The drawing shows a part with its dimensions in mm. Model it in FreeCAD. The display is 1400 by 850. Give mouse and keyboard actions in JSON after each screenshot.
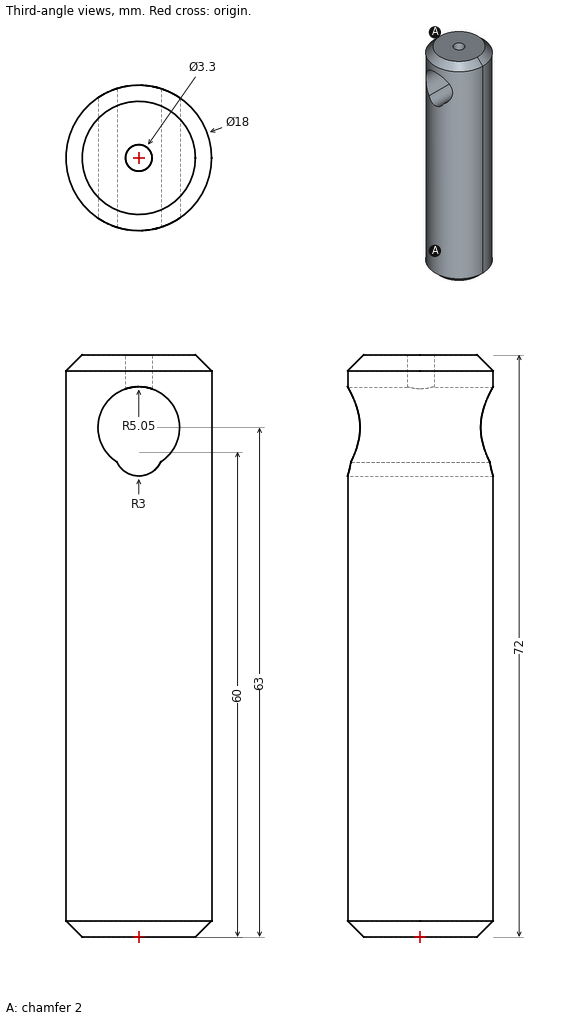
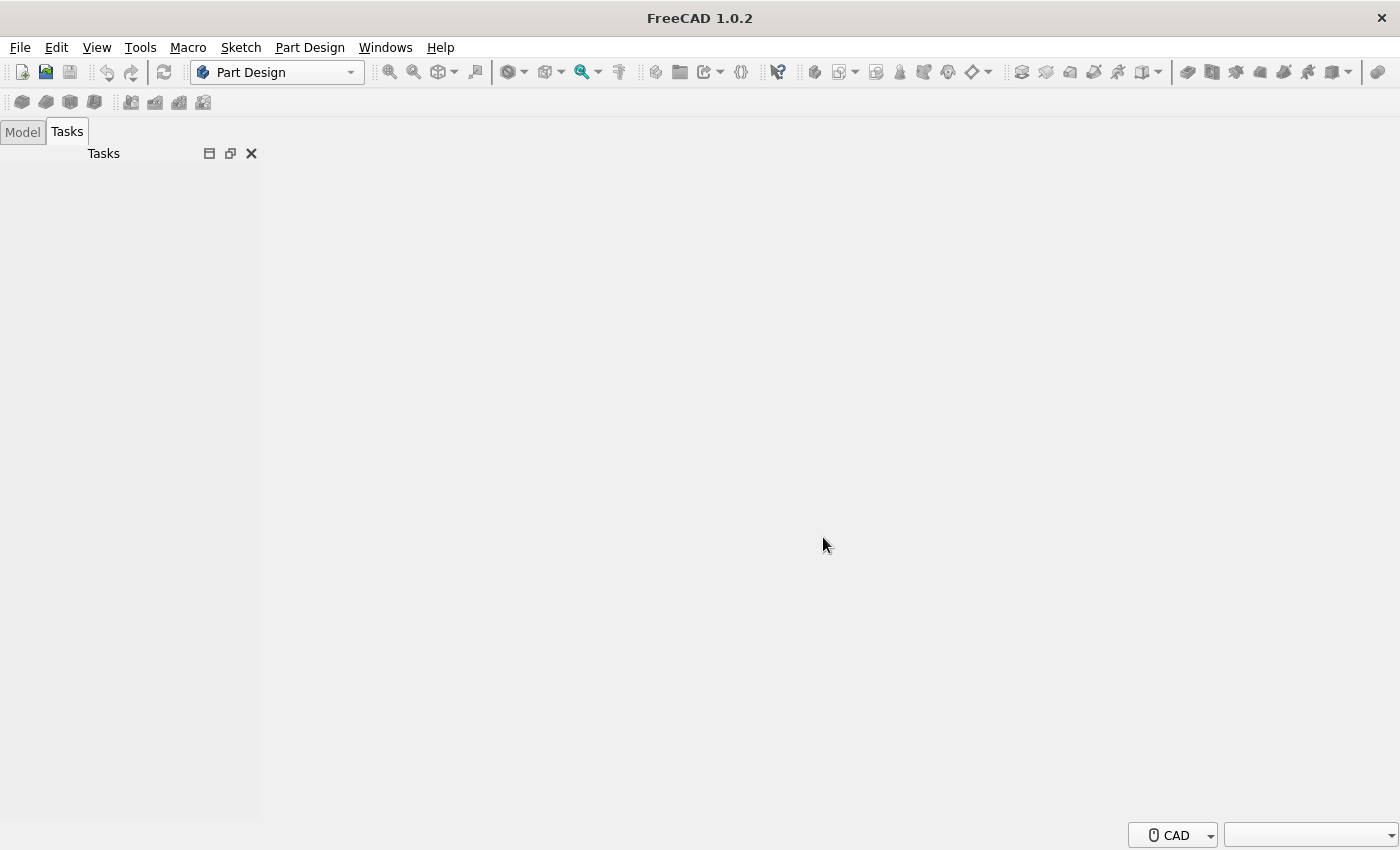
{"action": "key", "text": "ctrl+n"}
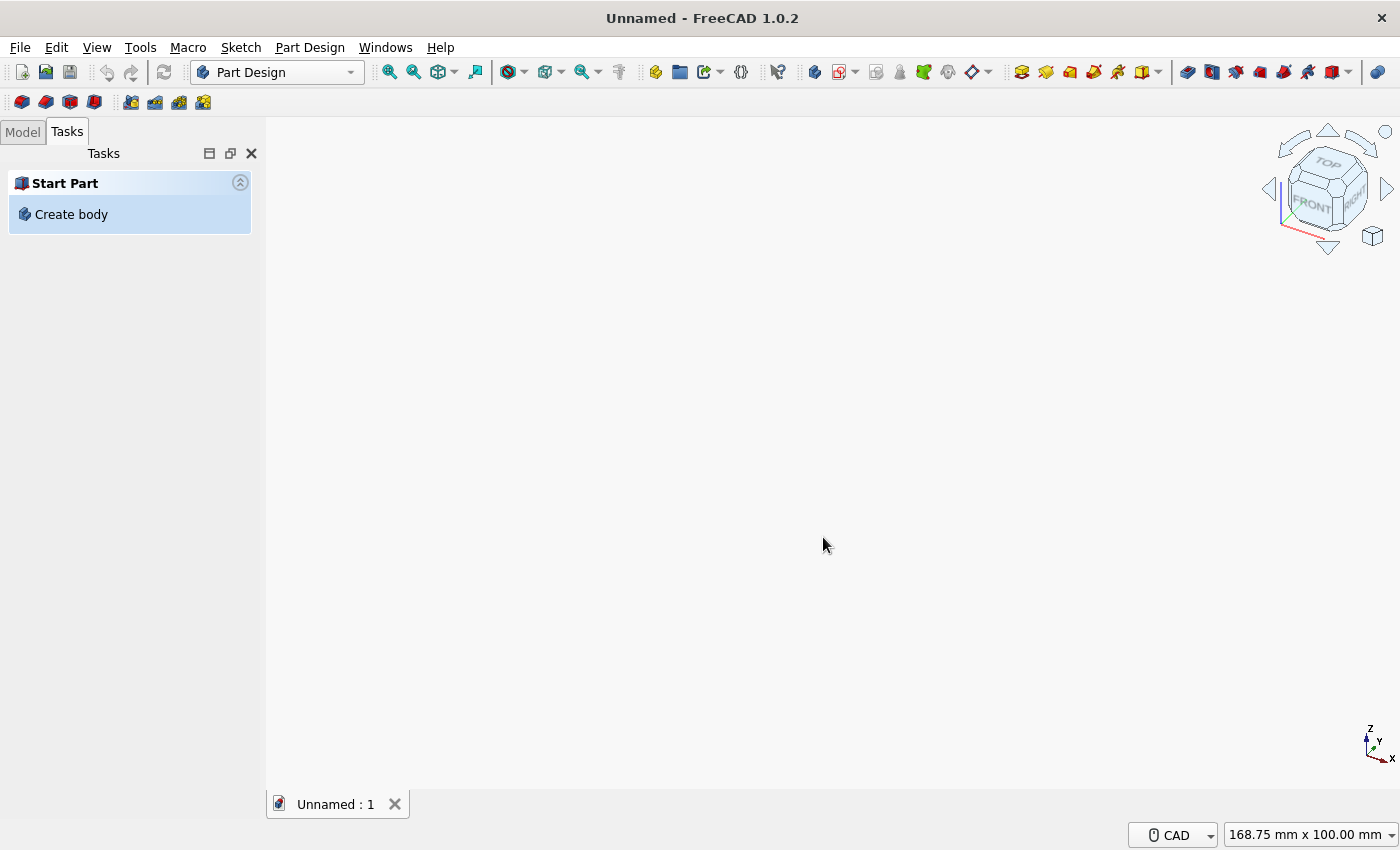
{"action": "left_click", "coordinate": [840, 72]}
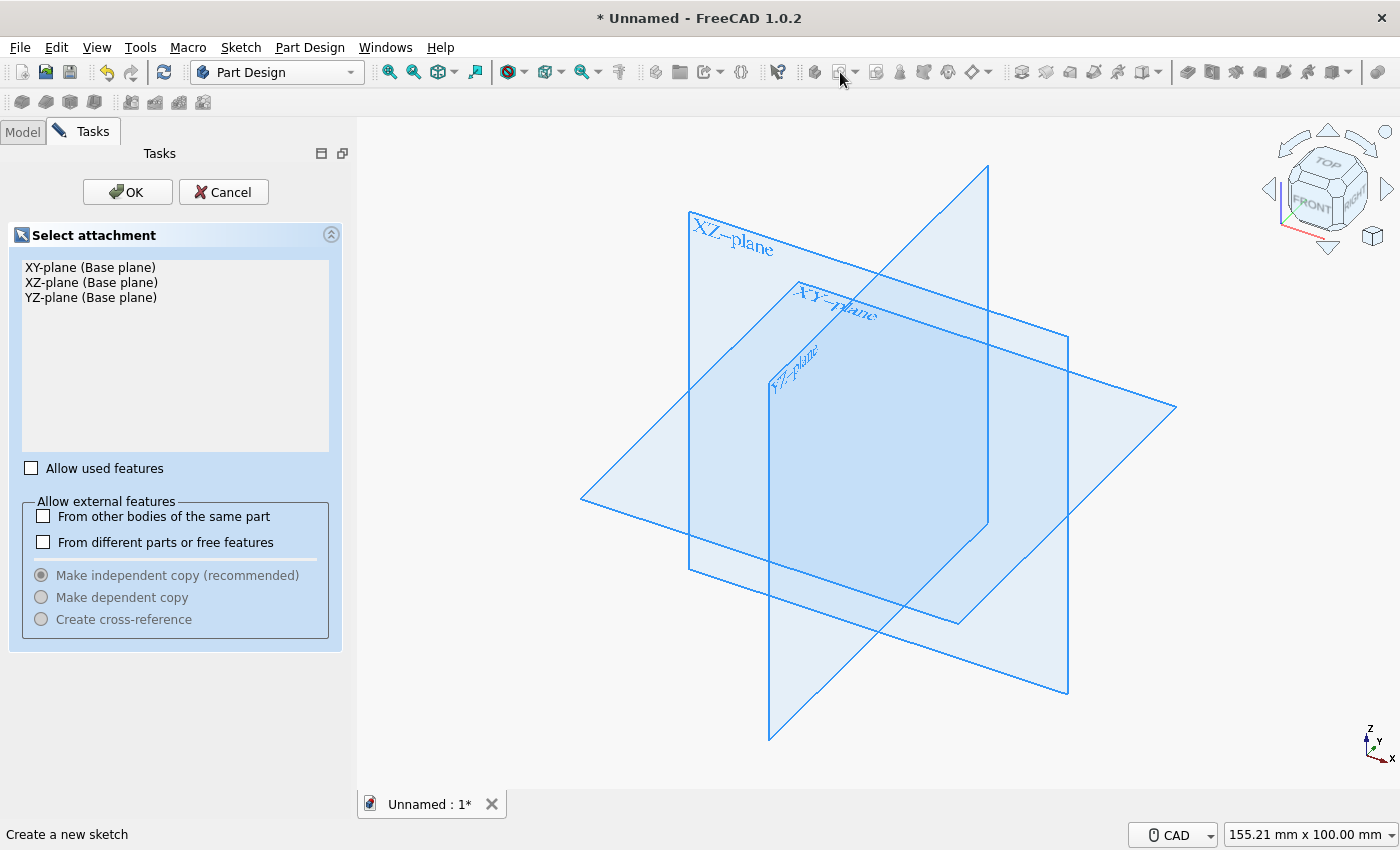
{"action": "left_click", "coordinate": [82, 268]}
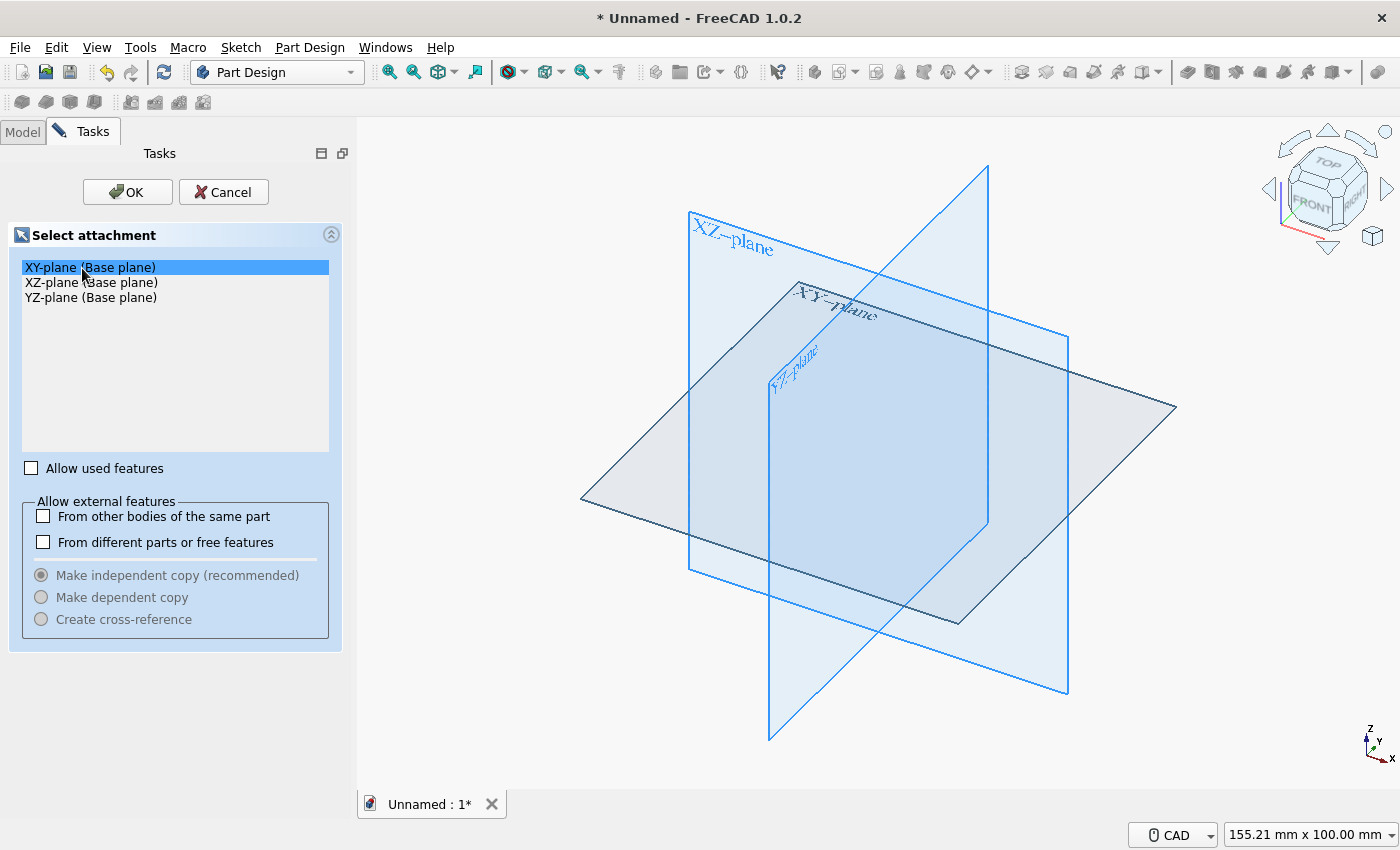
{"action": "left_click", "coordinate": [128, 192]}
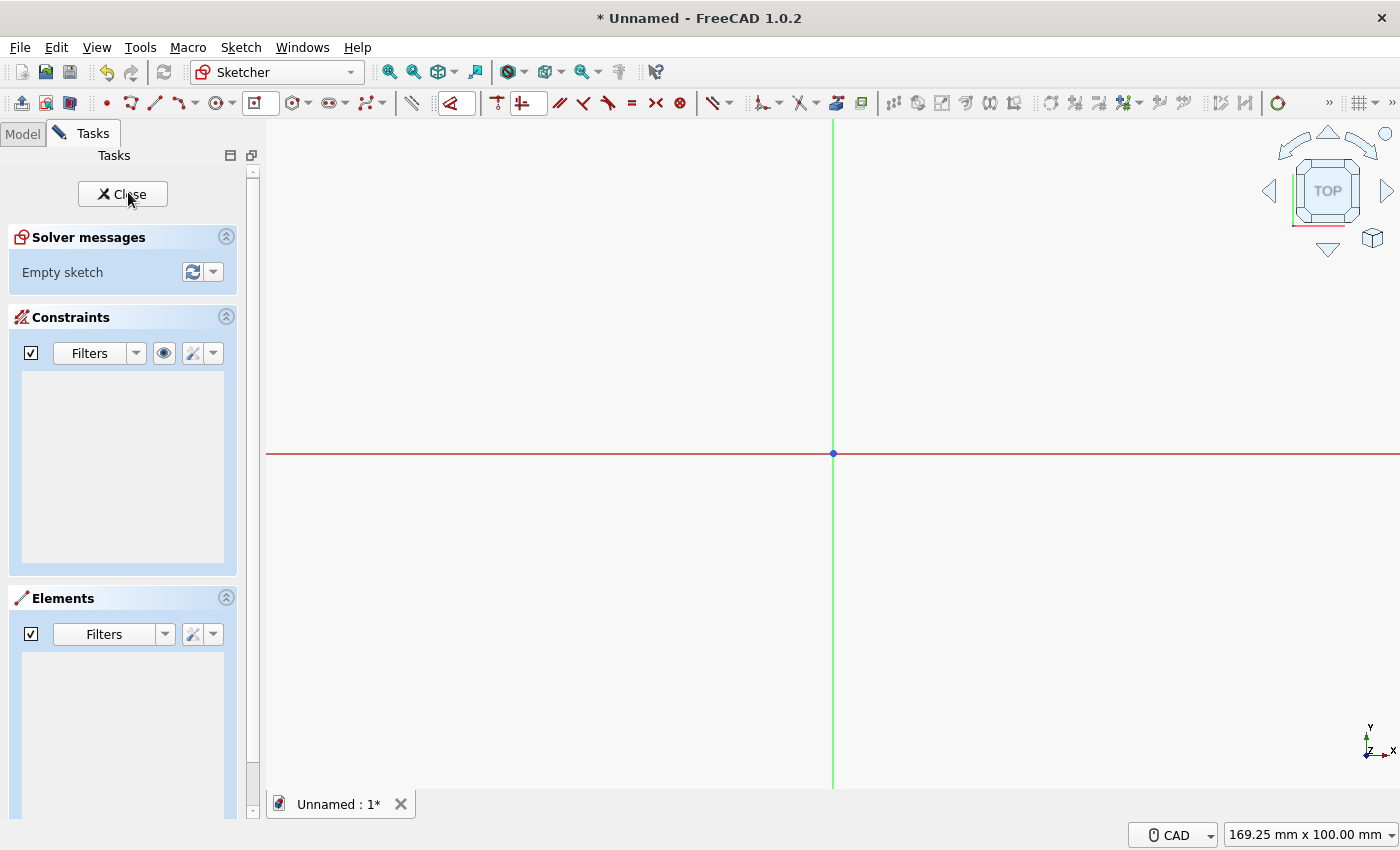
{"action": "scroll", "coordinate": [863, 454], "scroll_direction": "up", "scroll_amount": 6}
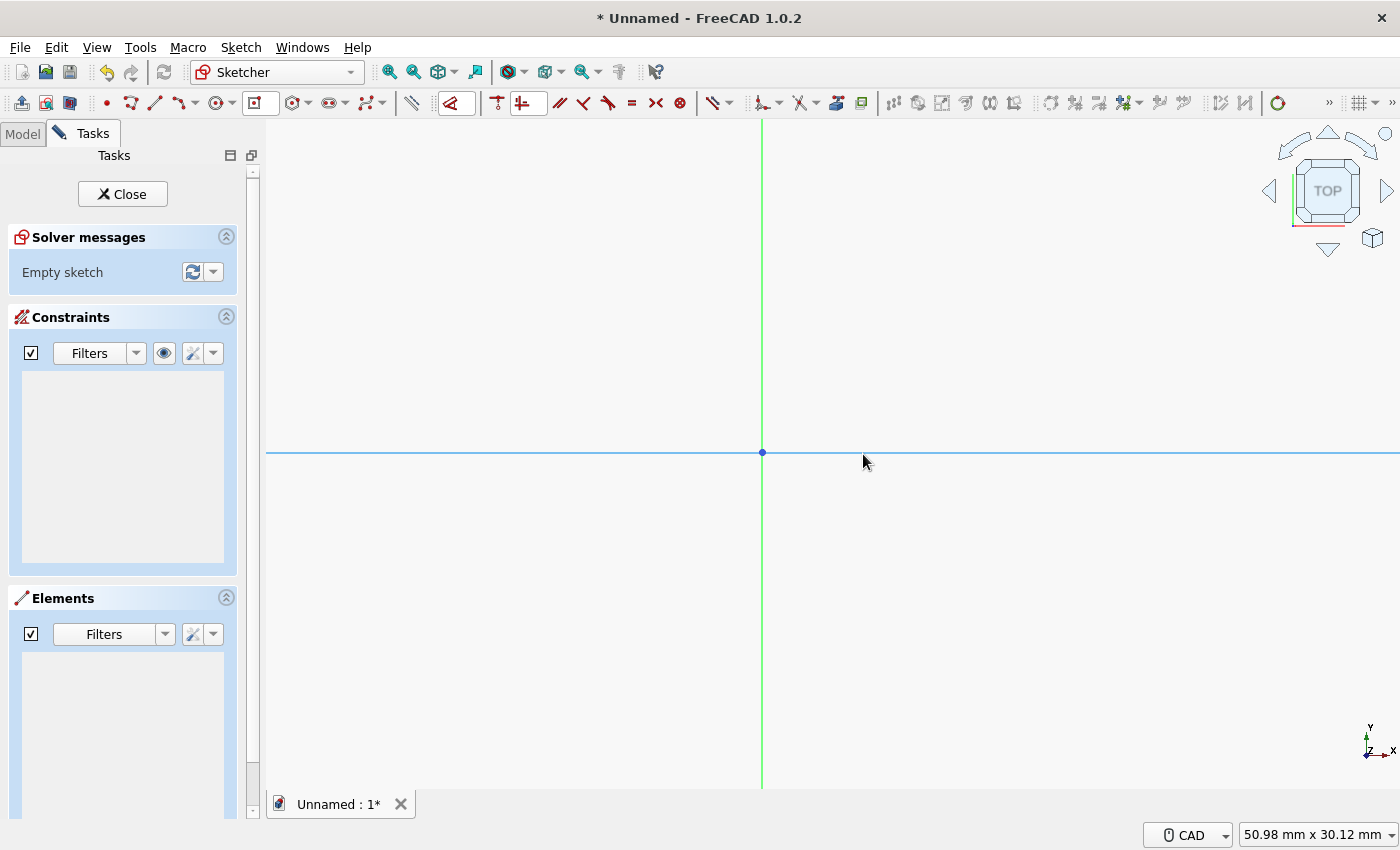
{"action": "key", "text": "g c"}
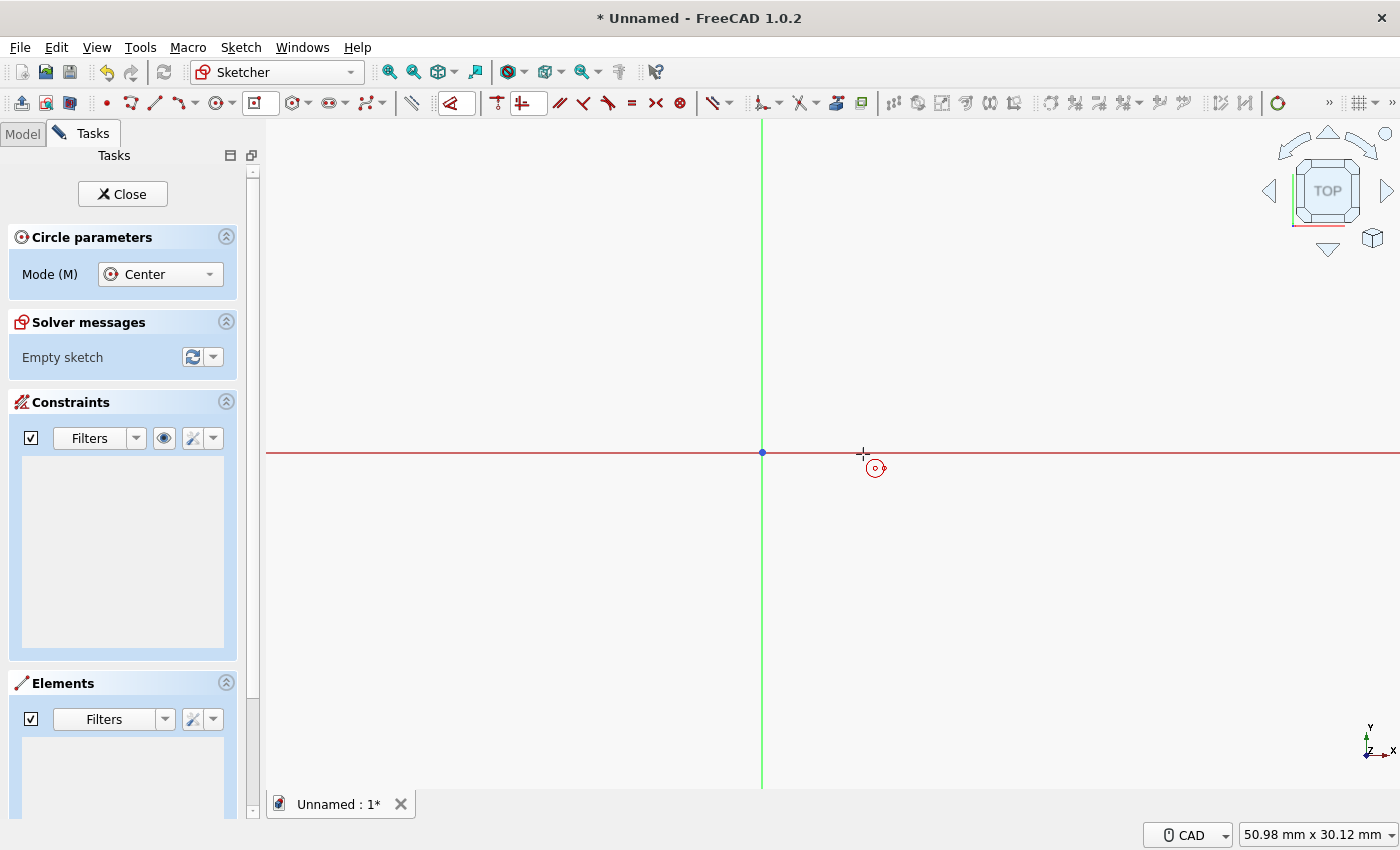
{"action": "left_click", "coordinate": [762, 453]}
{"action": "mouse_move", "coordinate": [904, 311]}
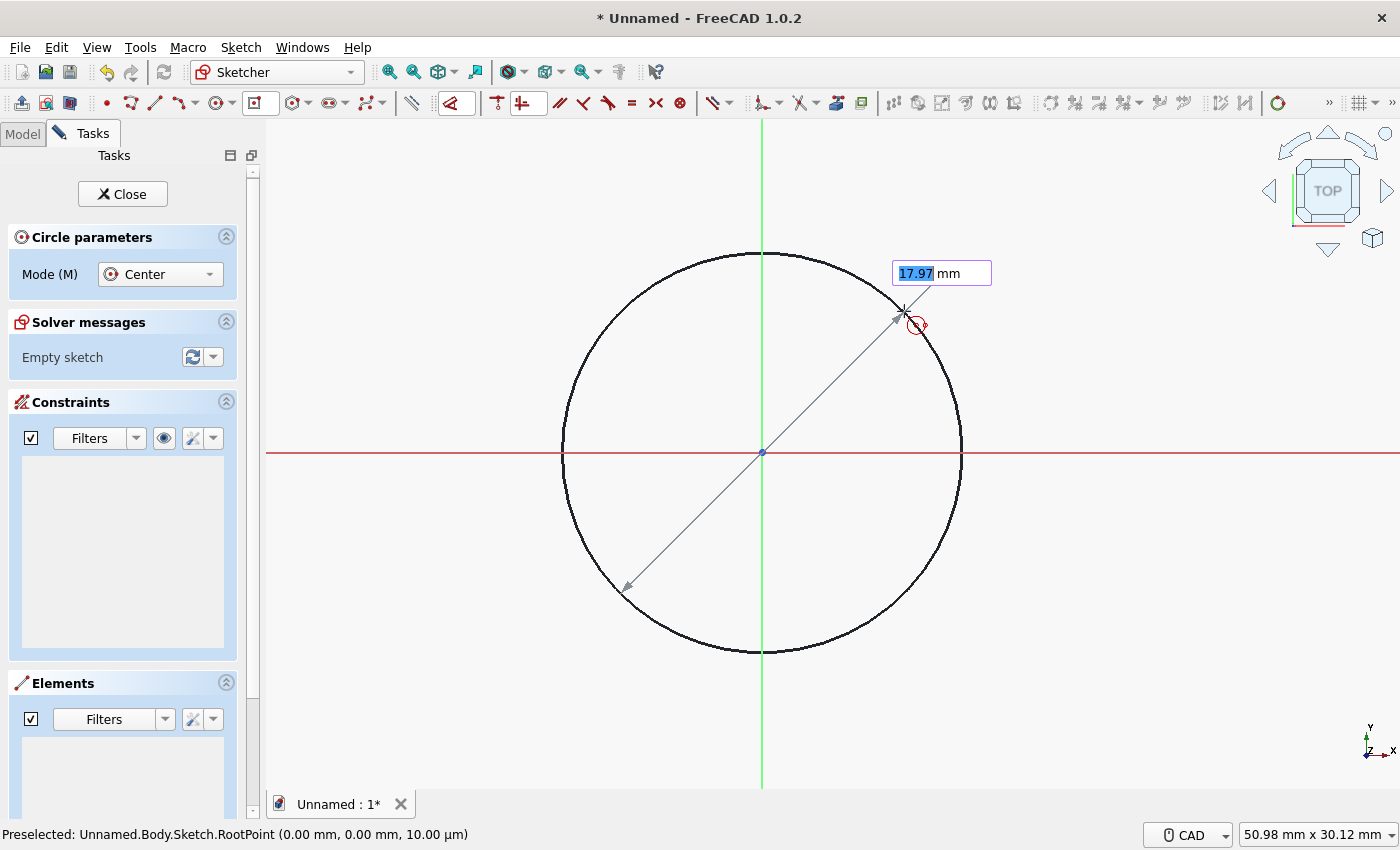
{"action": "type", "text": "18"}
{"action": "key", "text": "Return"}
{"action": "key", "text": "Escape"}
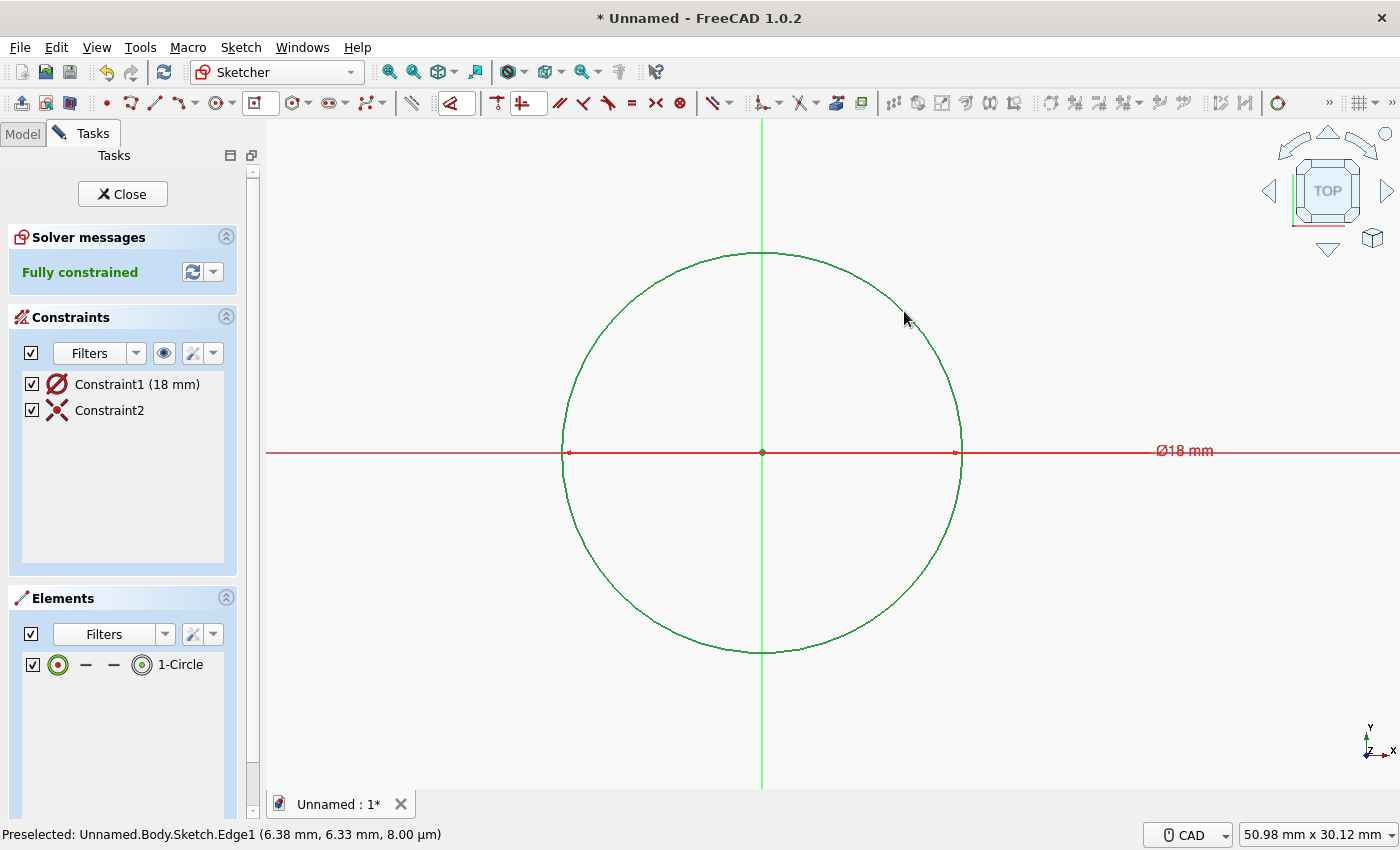
{"action": "left_click", "coordinate": [123, 194]}